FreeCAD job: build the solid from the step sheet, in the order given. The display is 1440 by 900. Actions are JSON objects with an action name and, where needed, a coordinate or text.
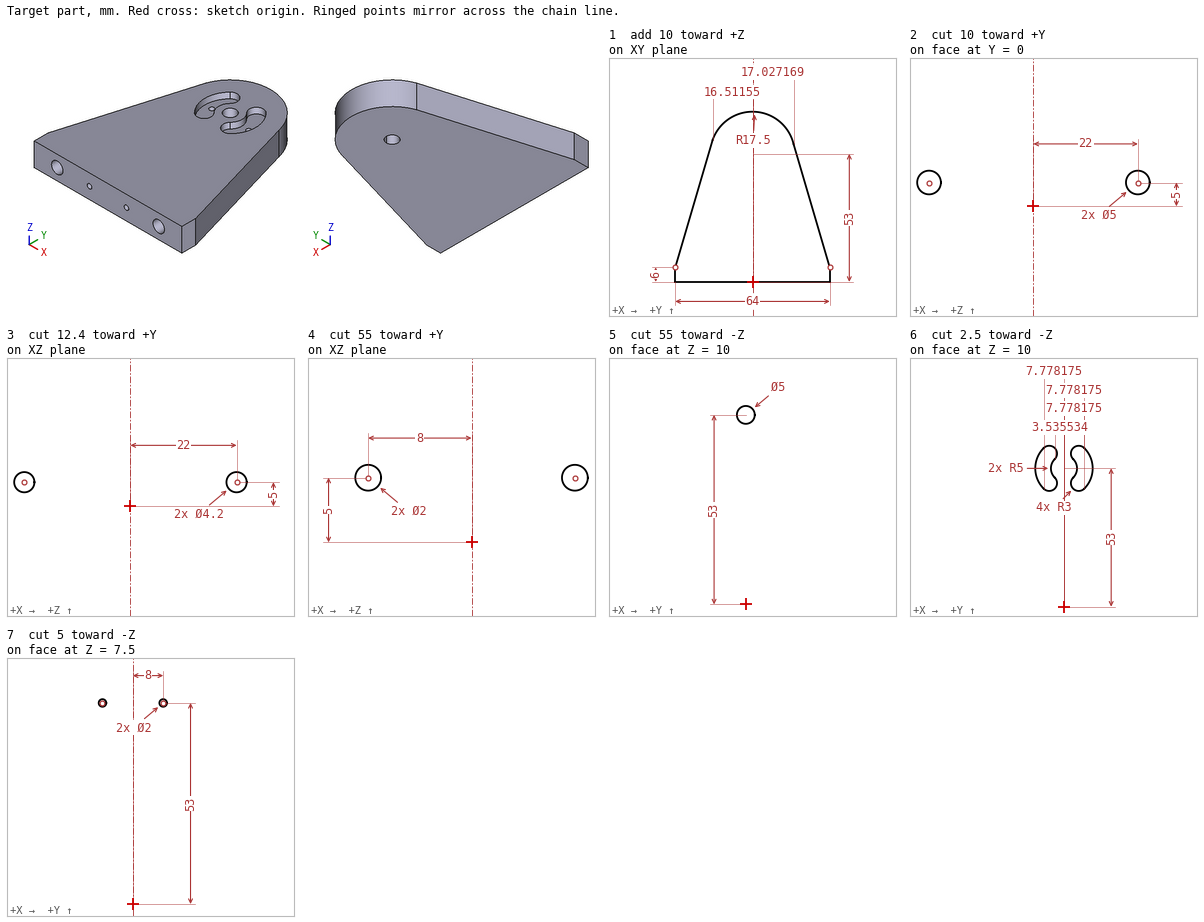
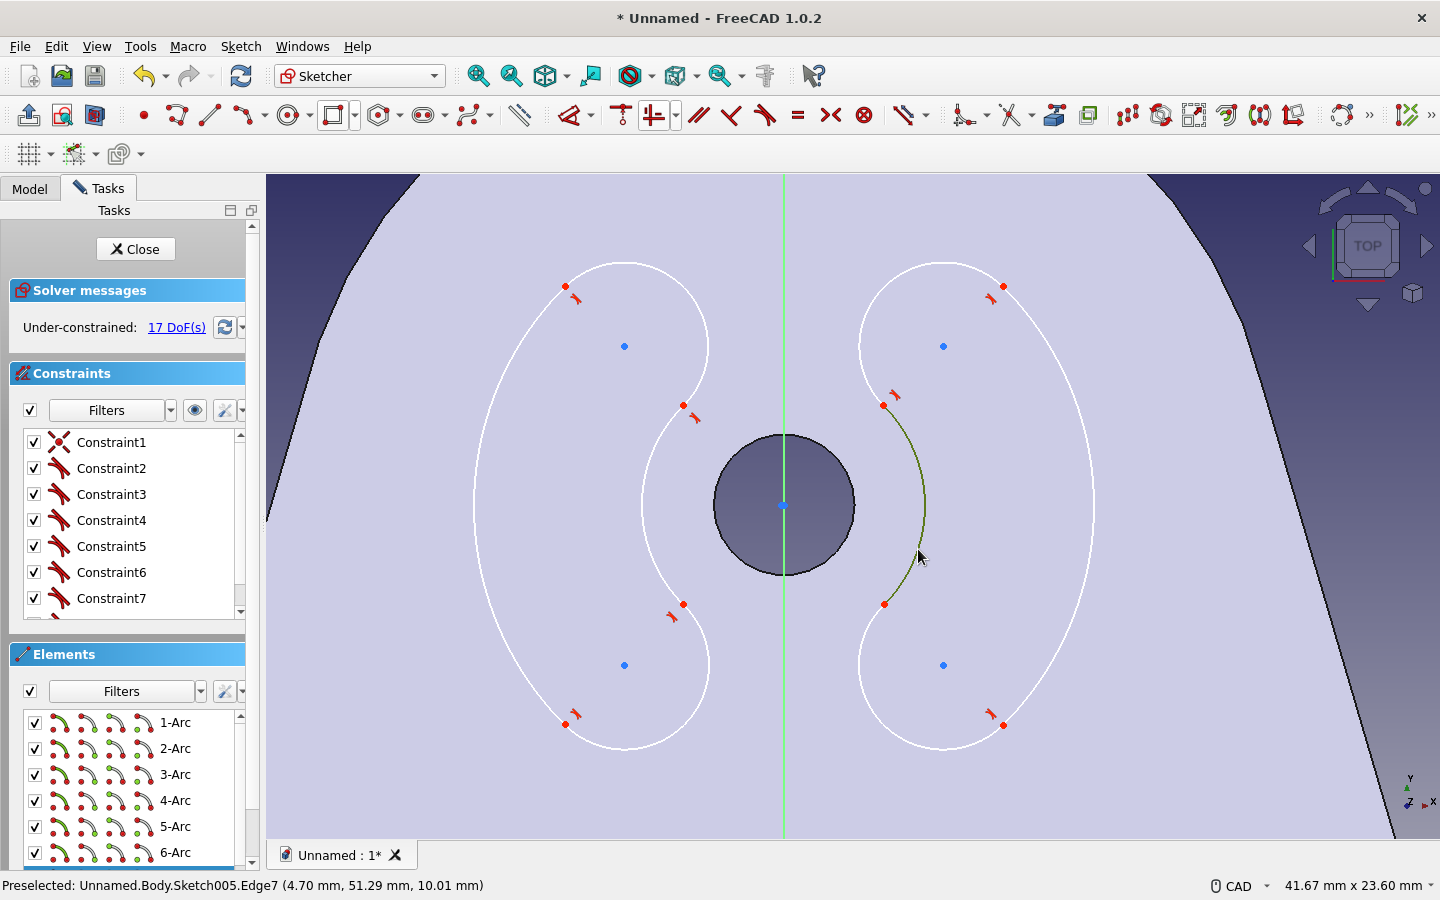
{"action": "left_click", "coordinate": [860, 678]}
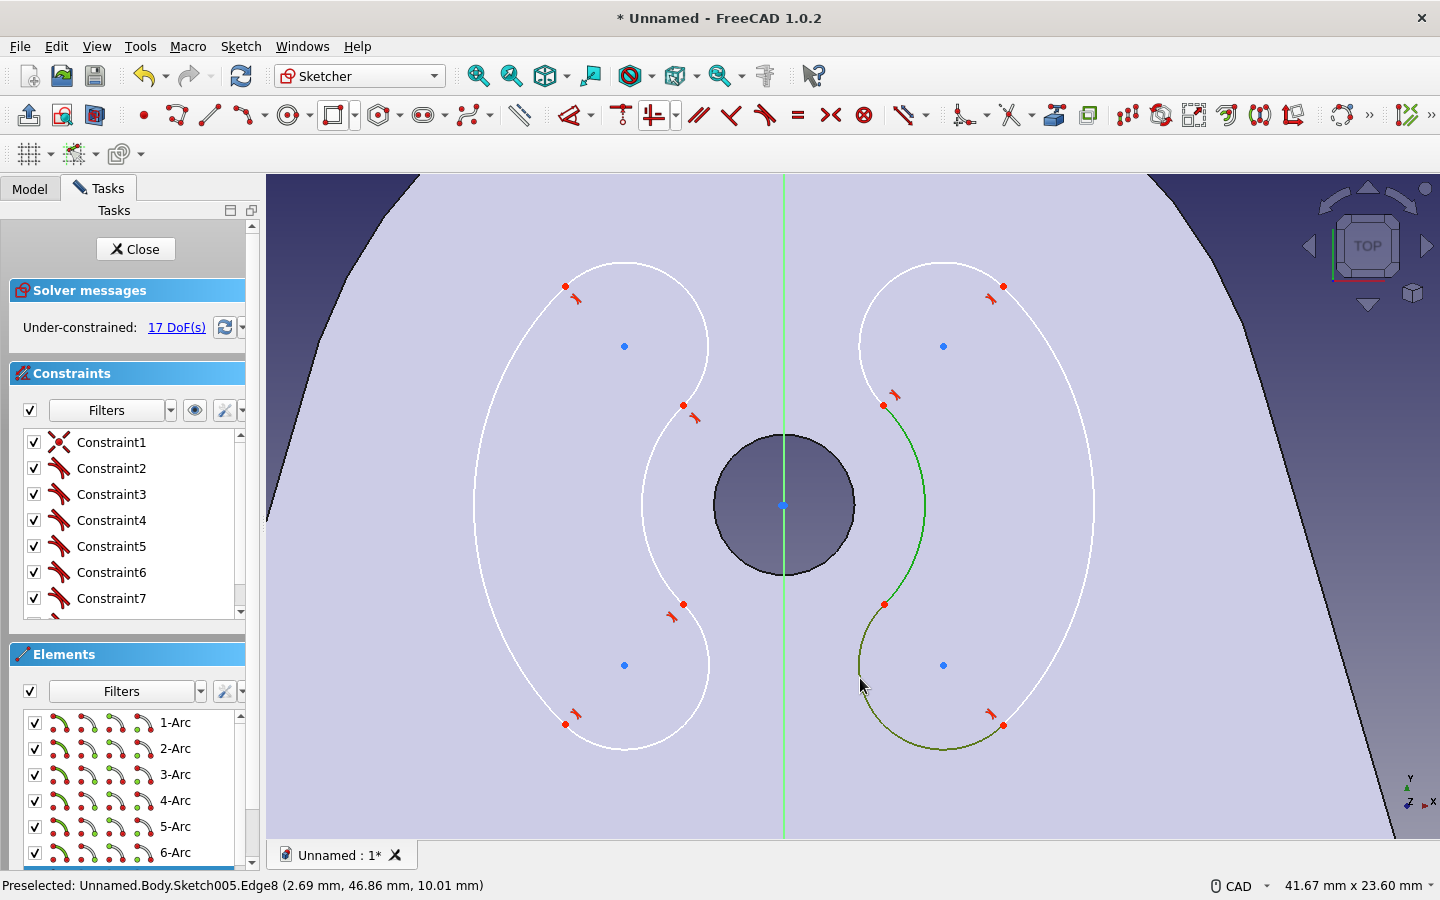
{"action": "left_click", "coordinate": [765, 116]}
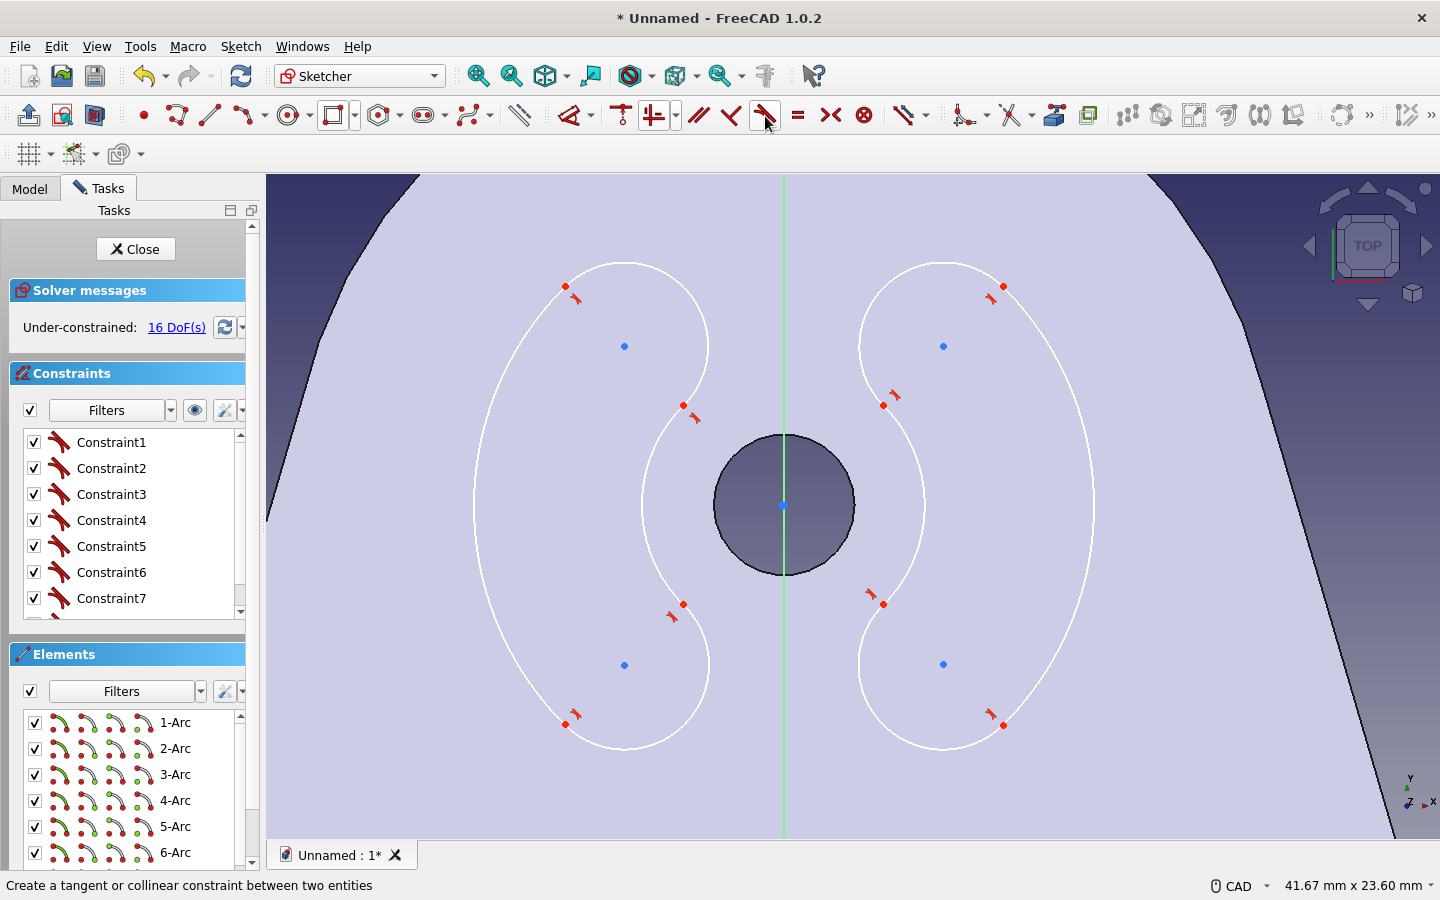
{"action": "left_click", "coordinate": [649, 462]}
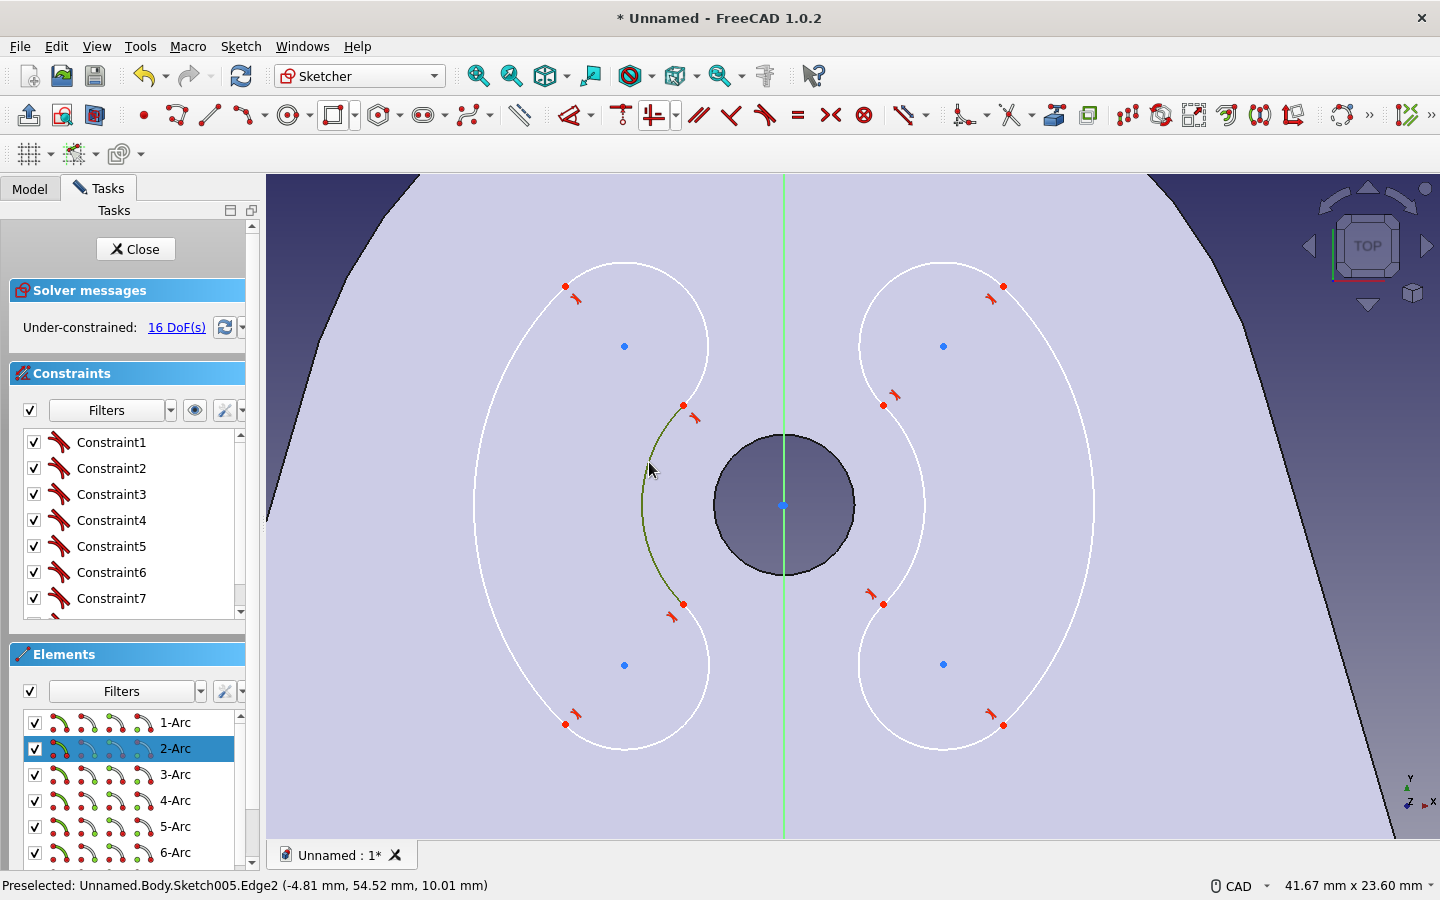
{"action": "left_click", "coordinate": [489, 410]}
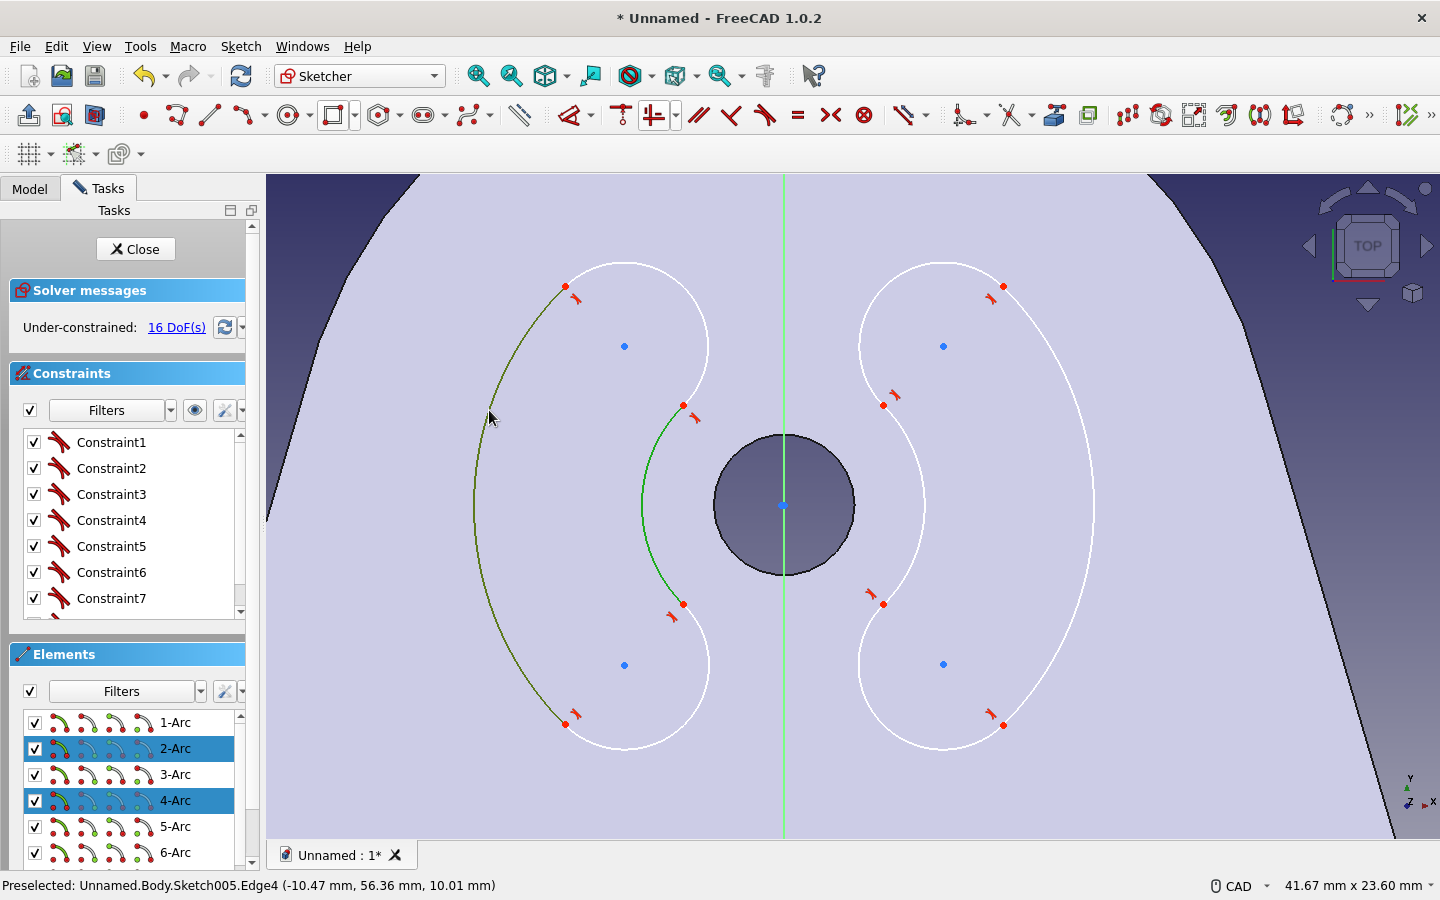
{"action": "left_click", "coordinate": [621, 116]}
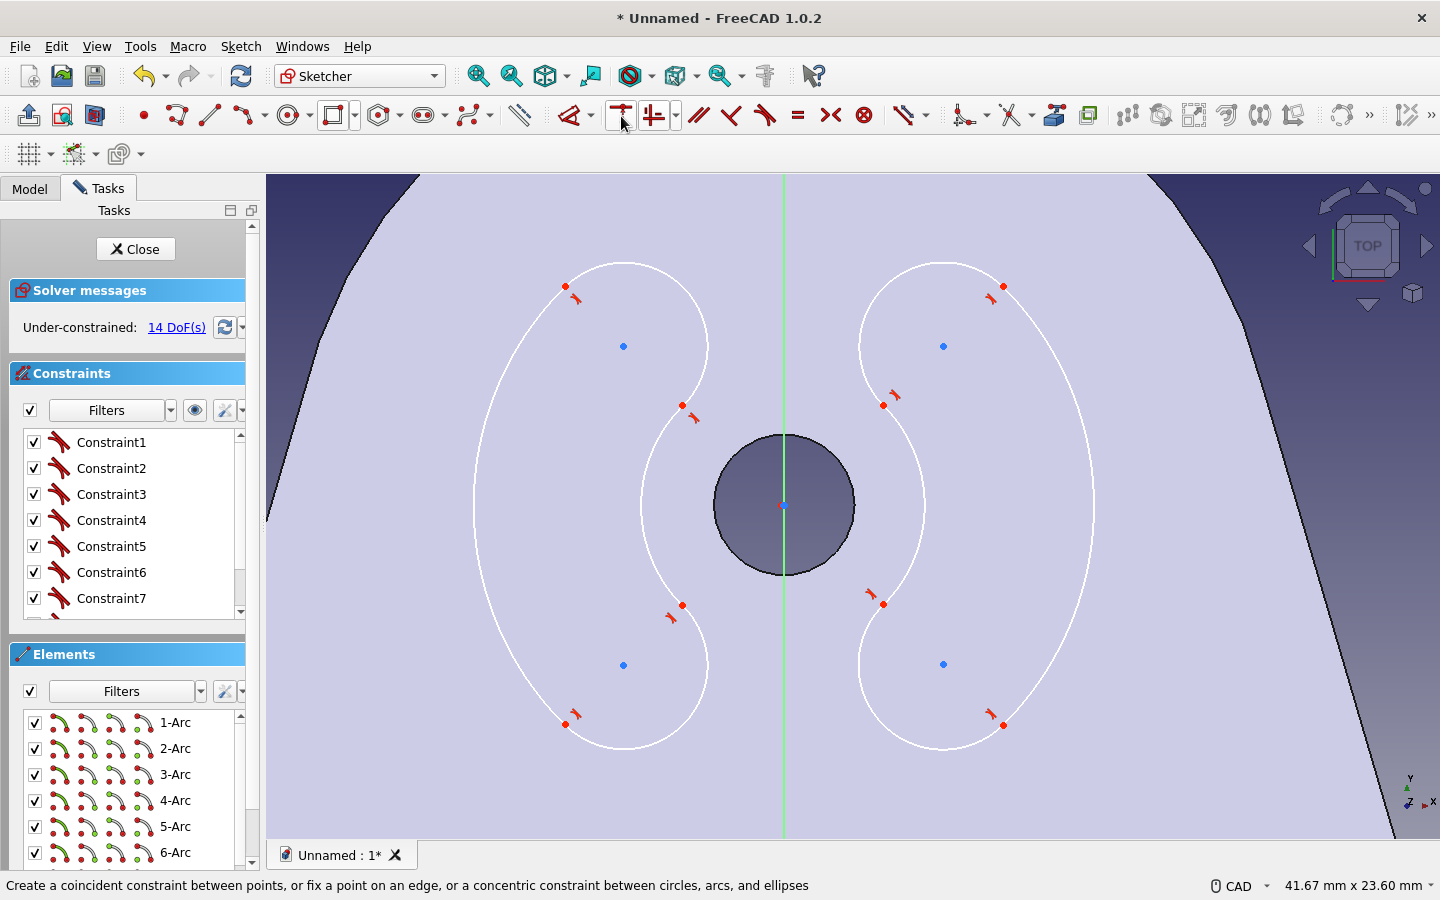
{"action": "left_click", "coordinate": [648, 462]}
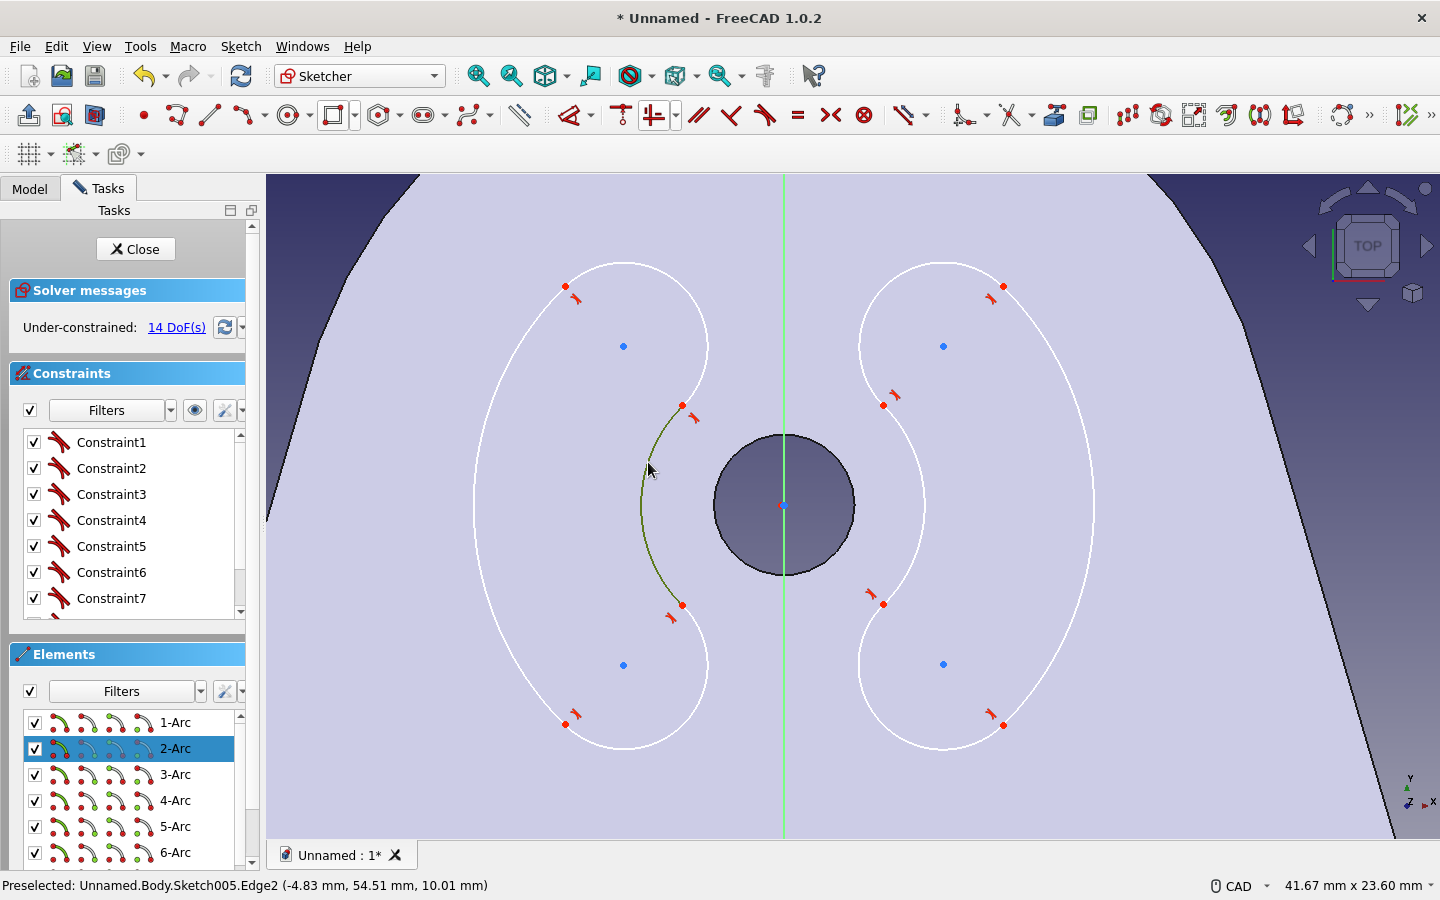
{"action": "left_click", "coordinate": [1079, 602]}